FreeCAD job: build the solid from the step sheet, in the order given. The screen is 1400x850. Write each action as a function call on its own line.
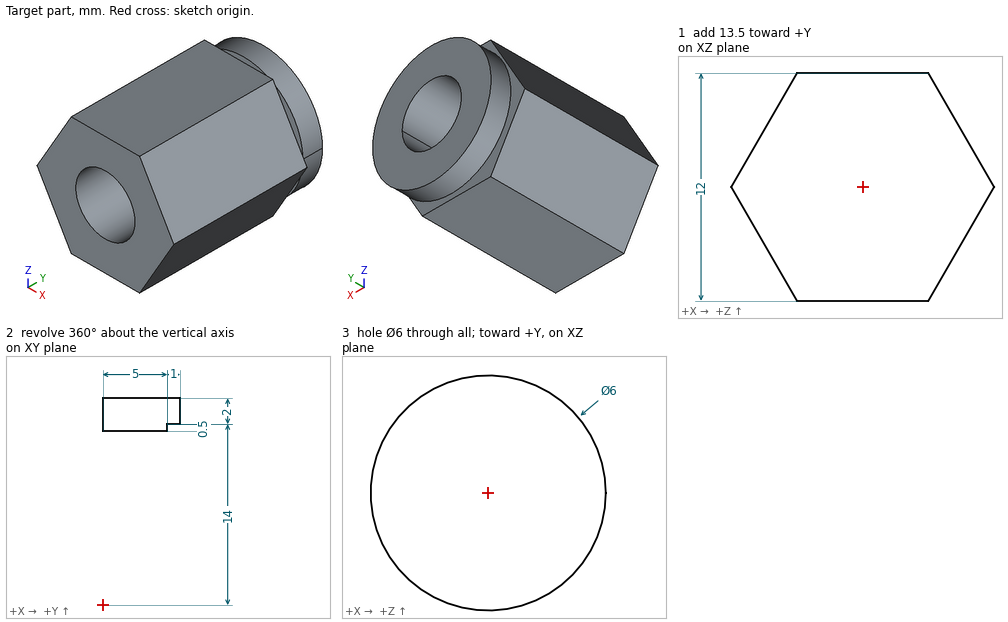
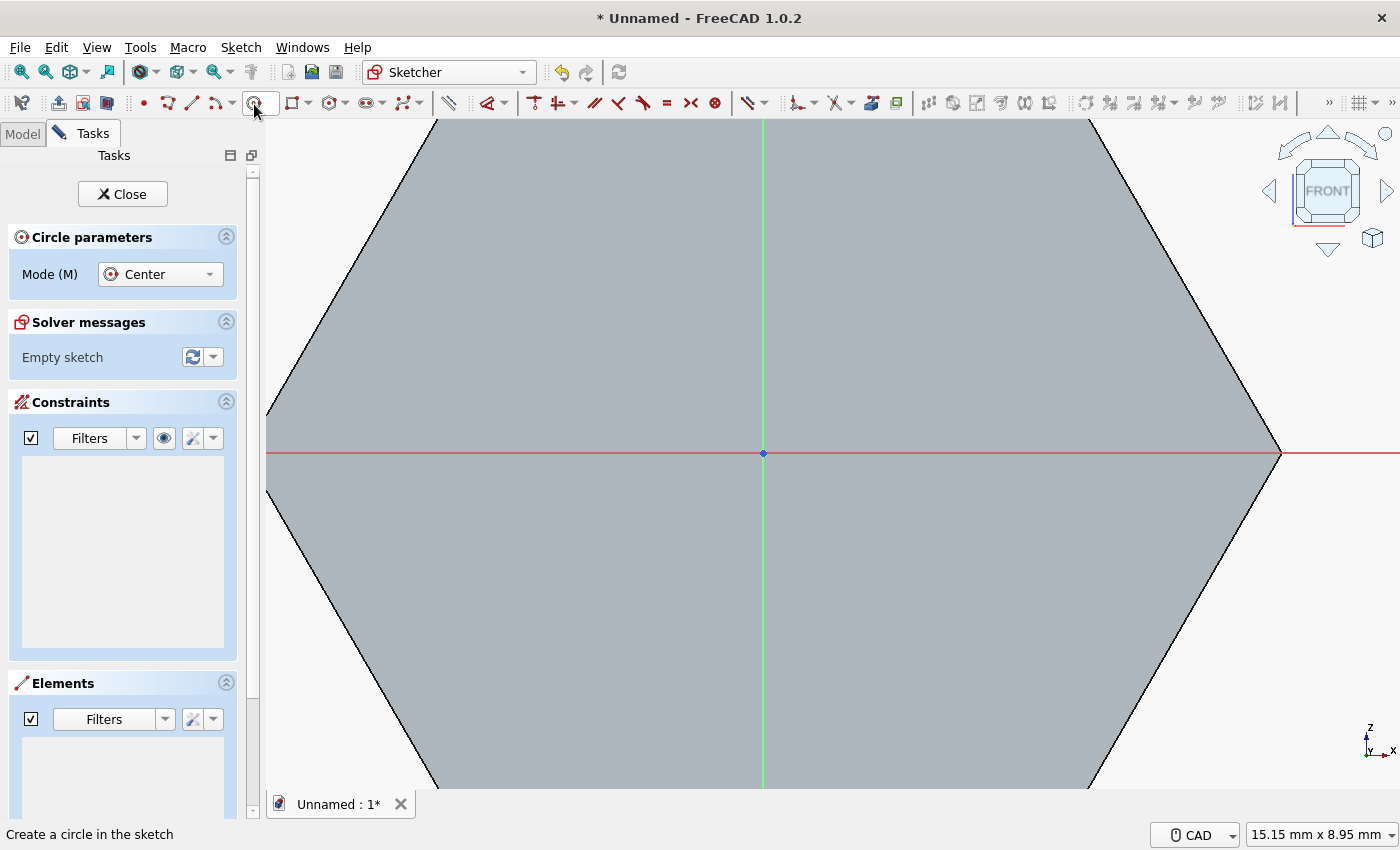
click(763, 453)
move(922, 294)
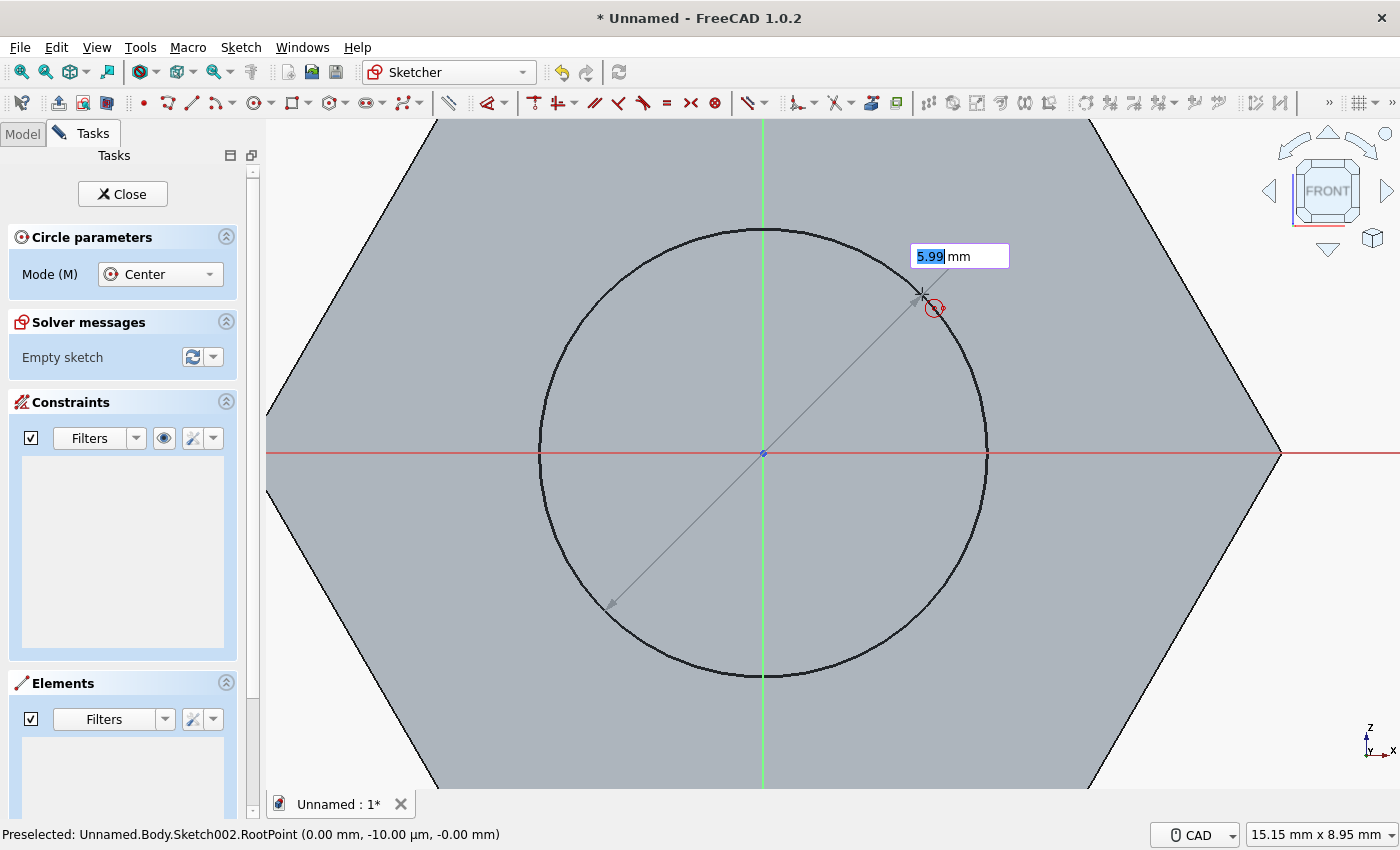
text(6)
key(Return)
key(Escape)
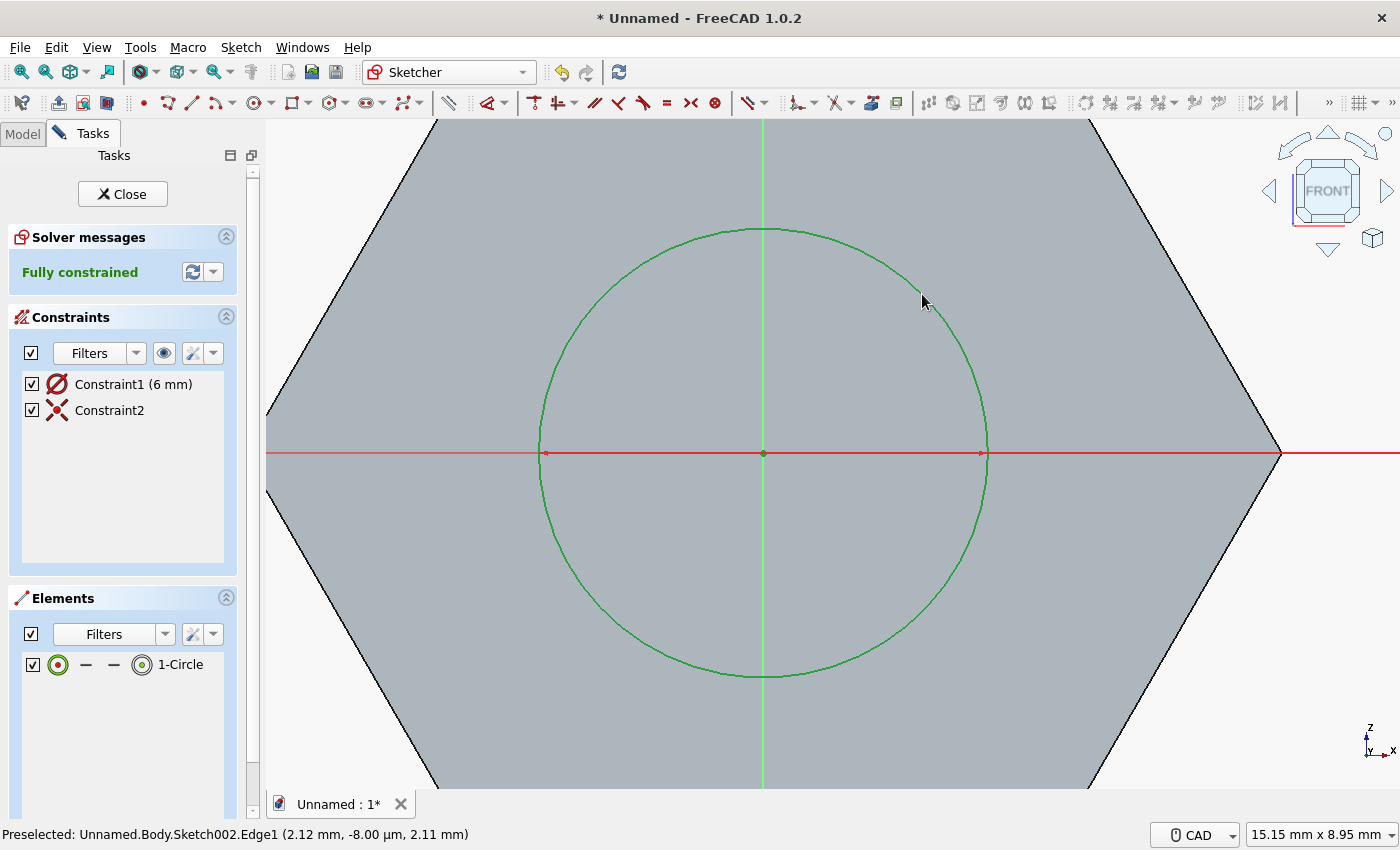
click(123, 194)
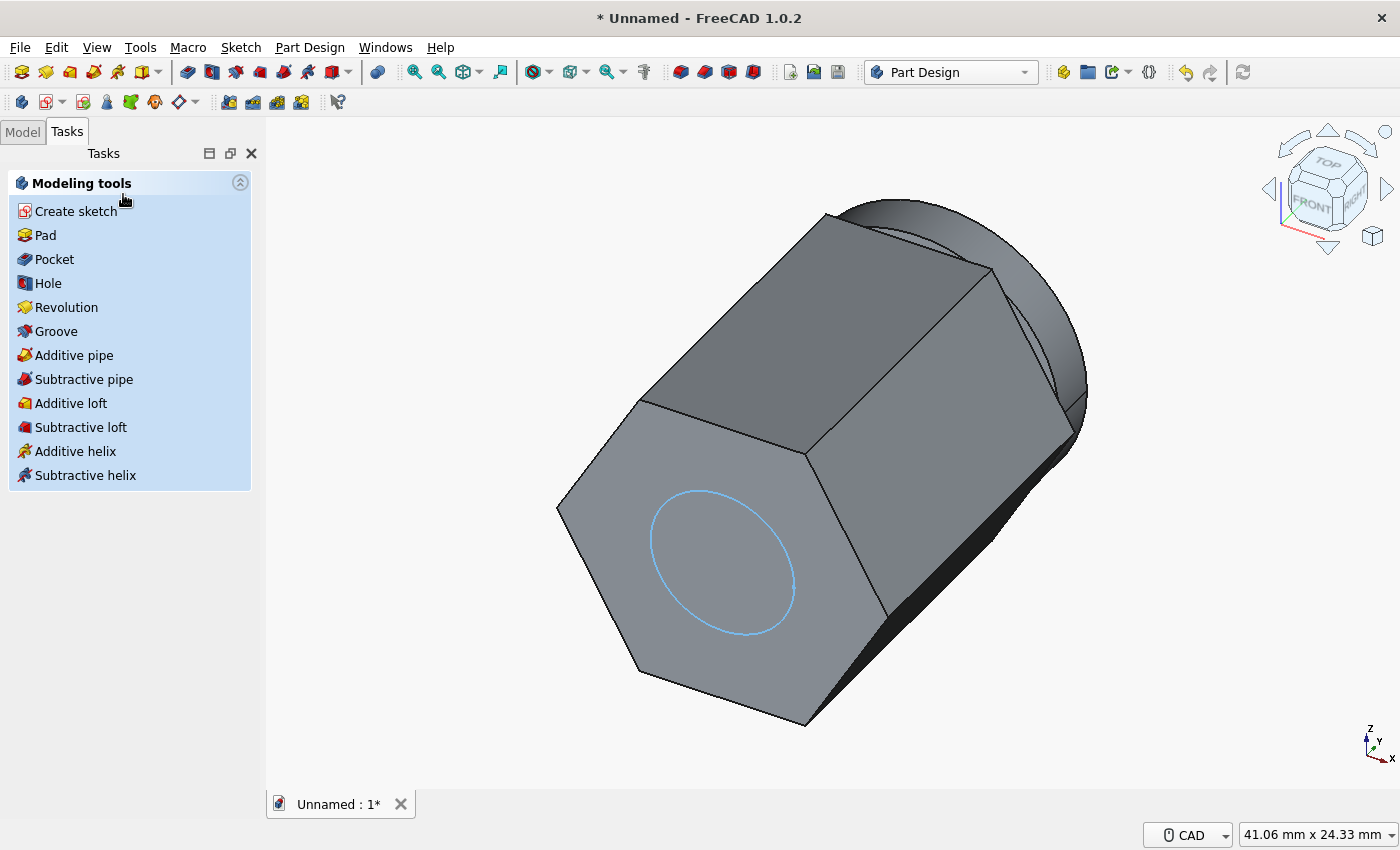
click(212, 72)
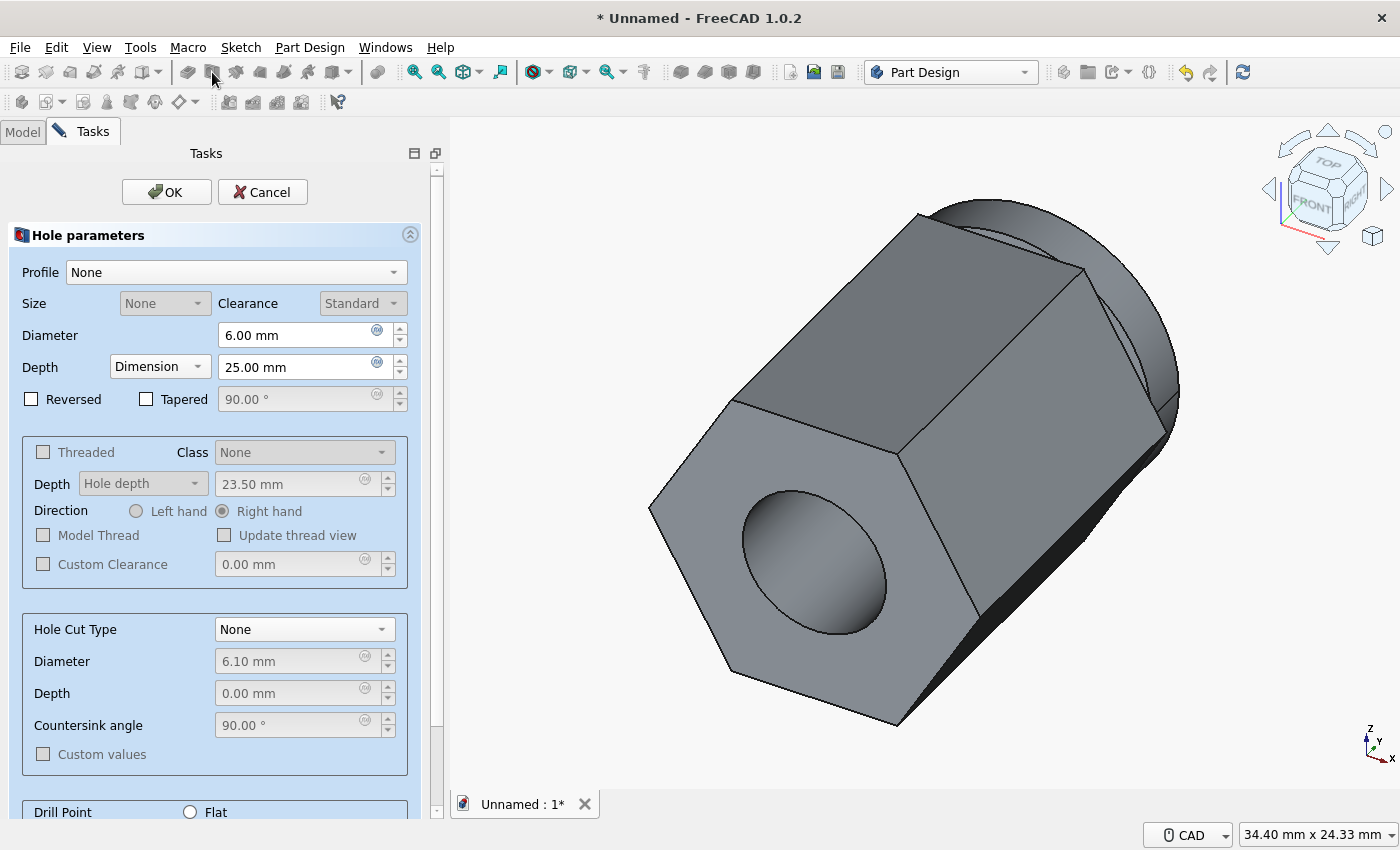
triple_click(305, 335)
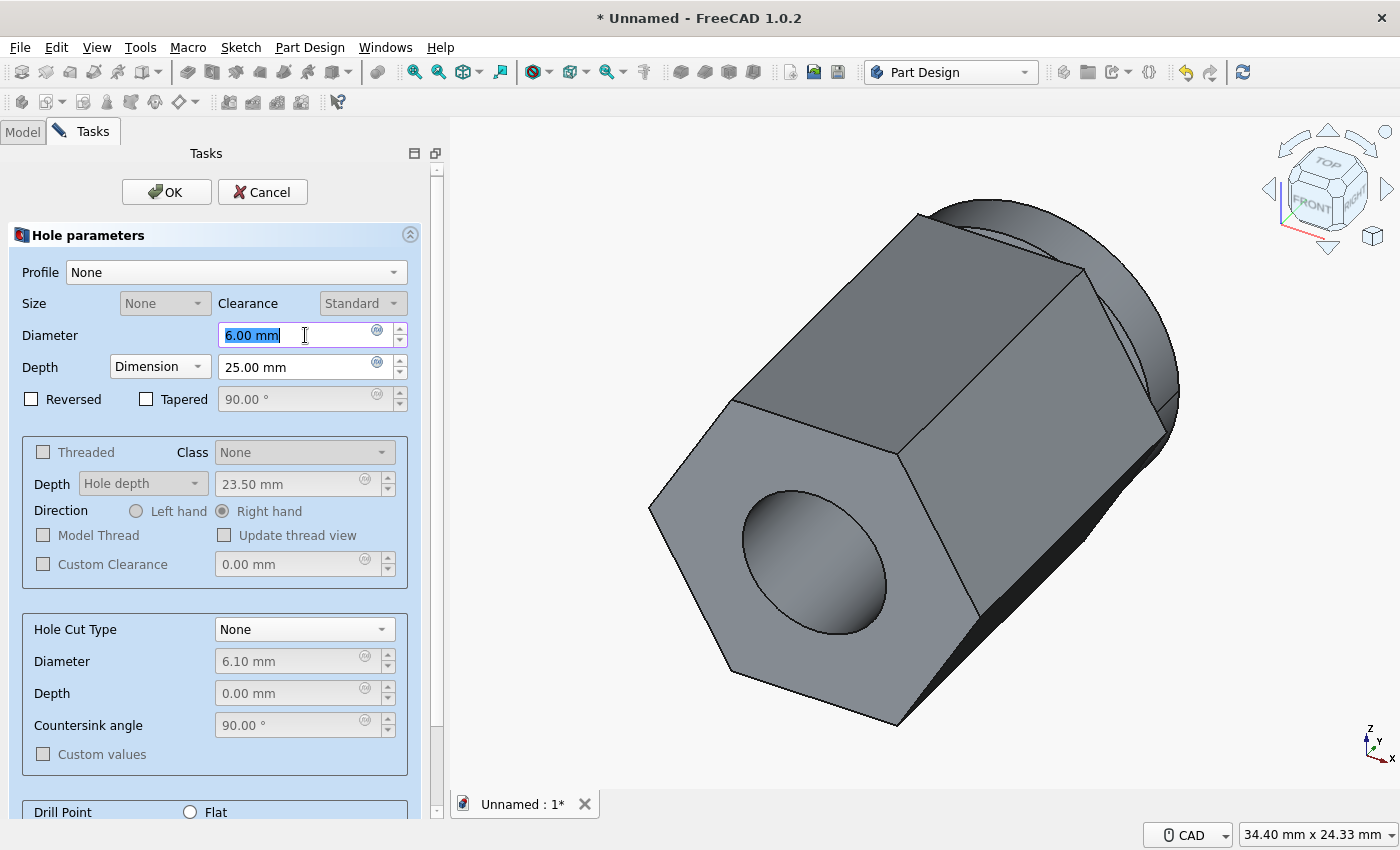
text(6)
key(Tab)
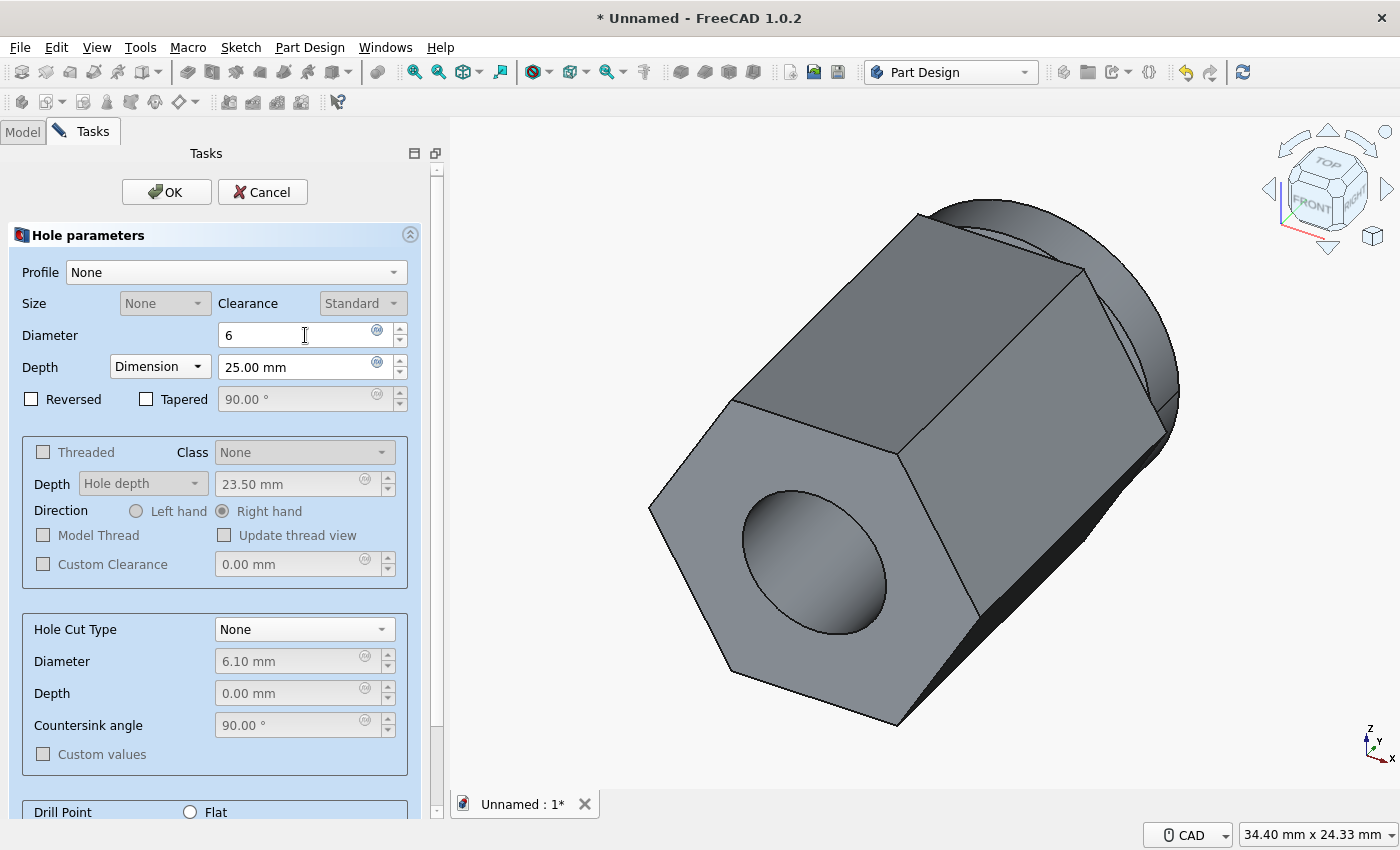
click(161, 366)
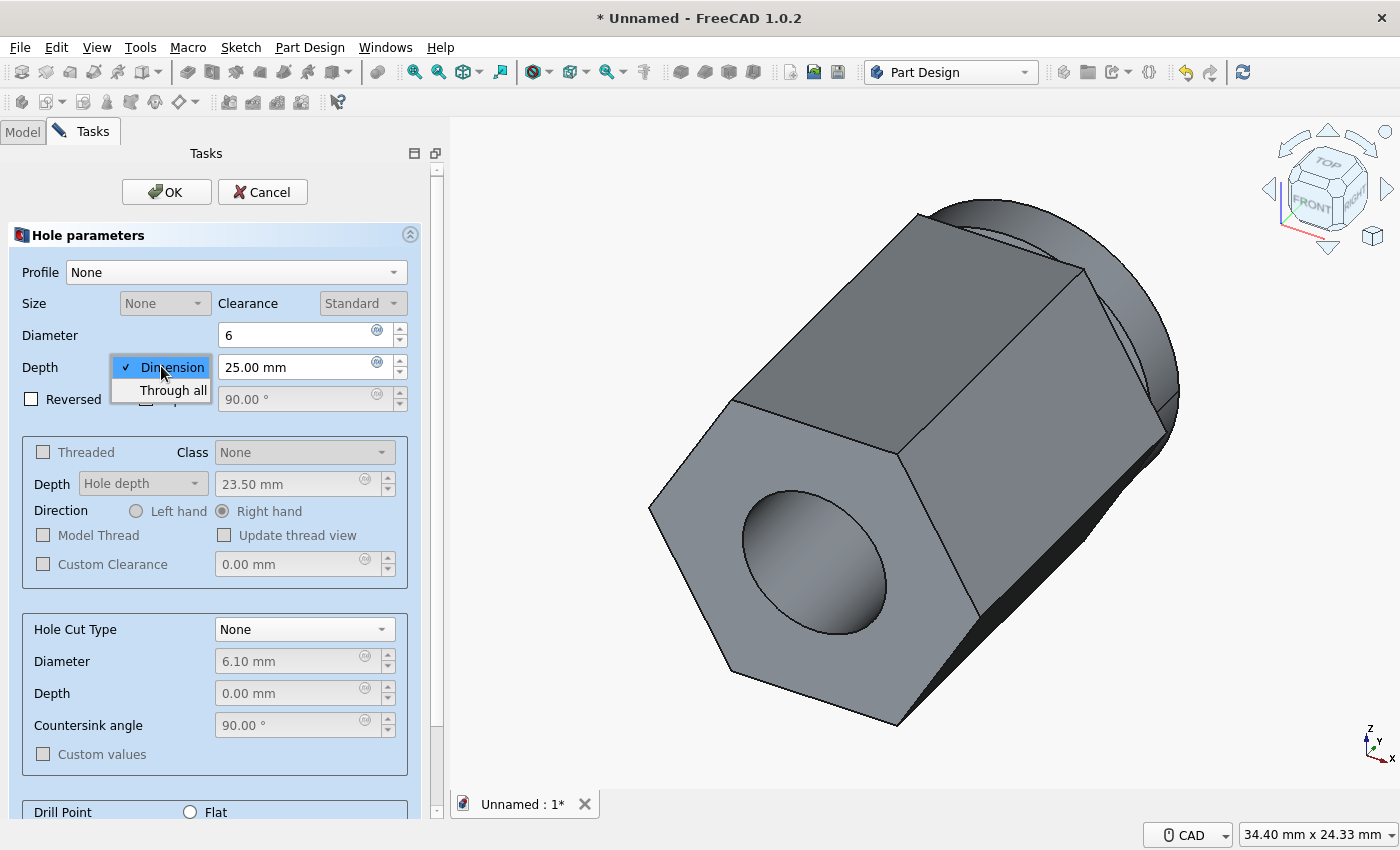
click(160, 390)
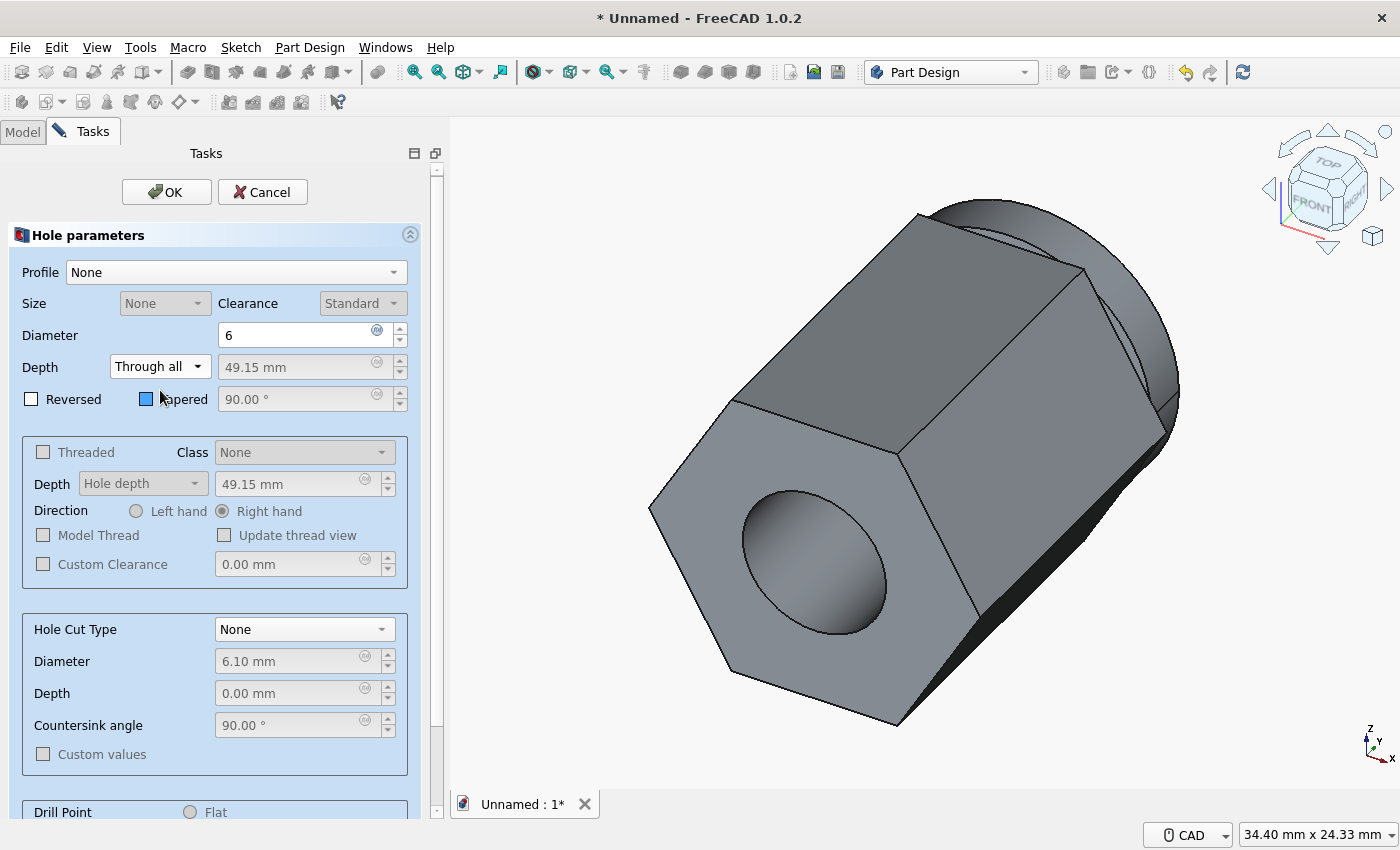
click(167, 192)